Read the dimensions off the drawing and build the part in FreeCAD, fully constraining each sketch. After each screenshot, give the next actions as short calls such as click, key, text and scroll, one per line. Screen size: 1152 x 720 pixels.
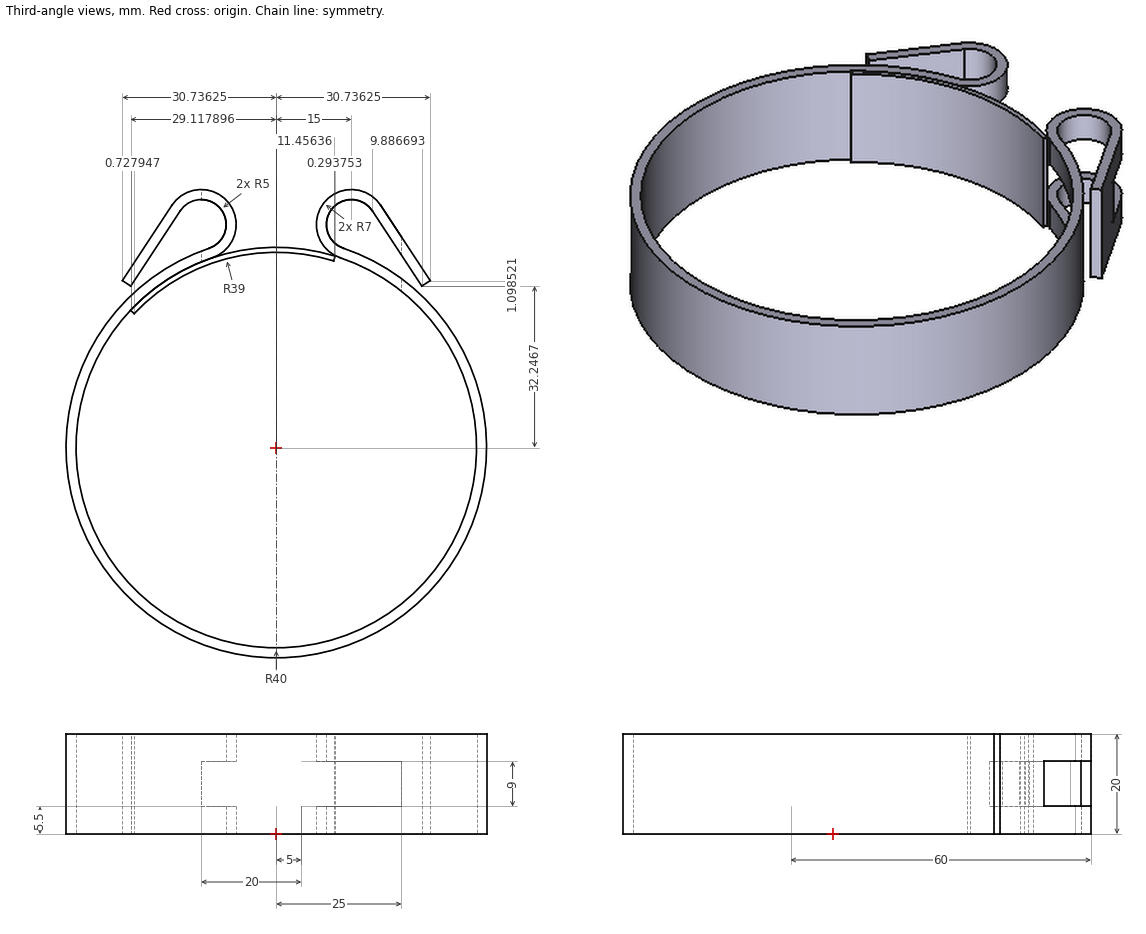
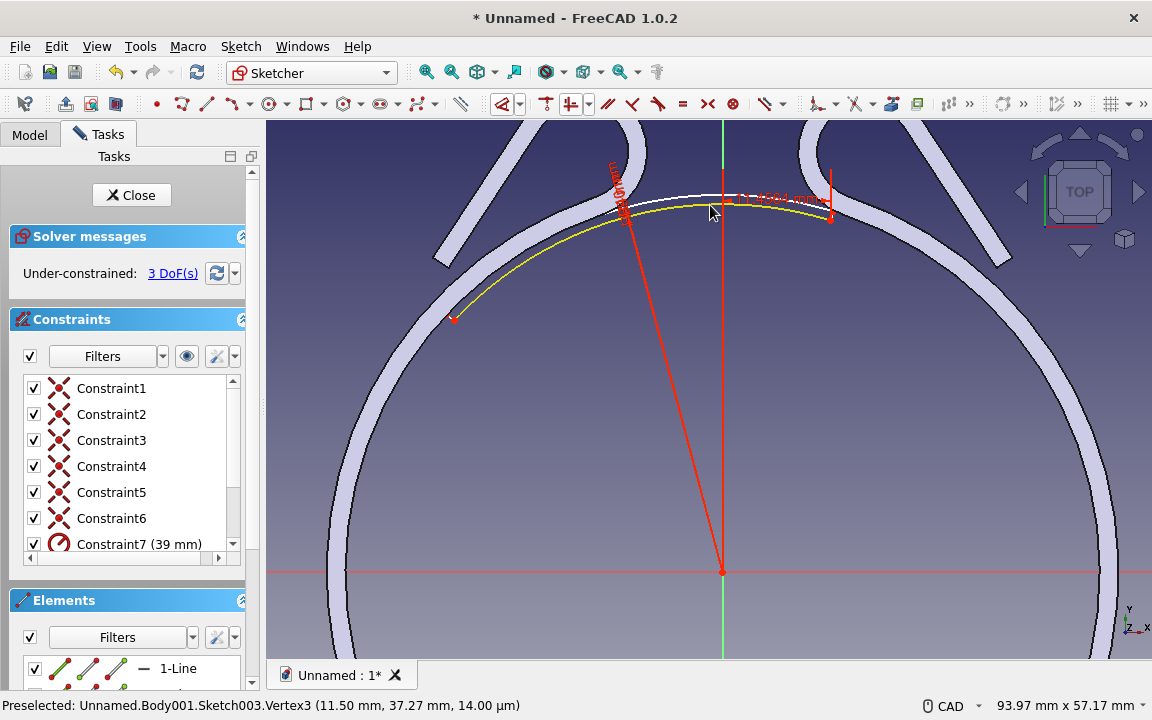
scroll(450, 318, up, 9)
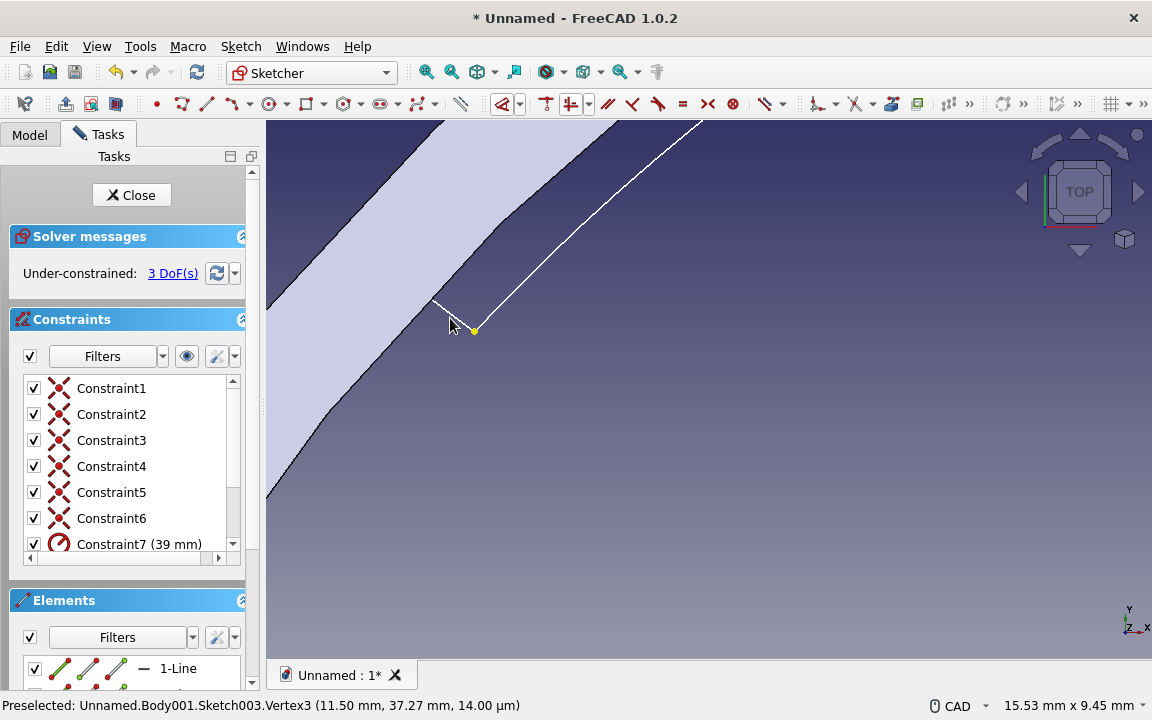
click(452, 315)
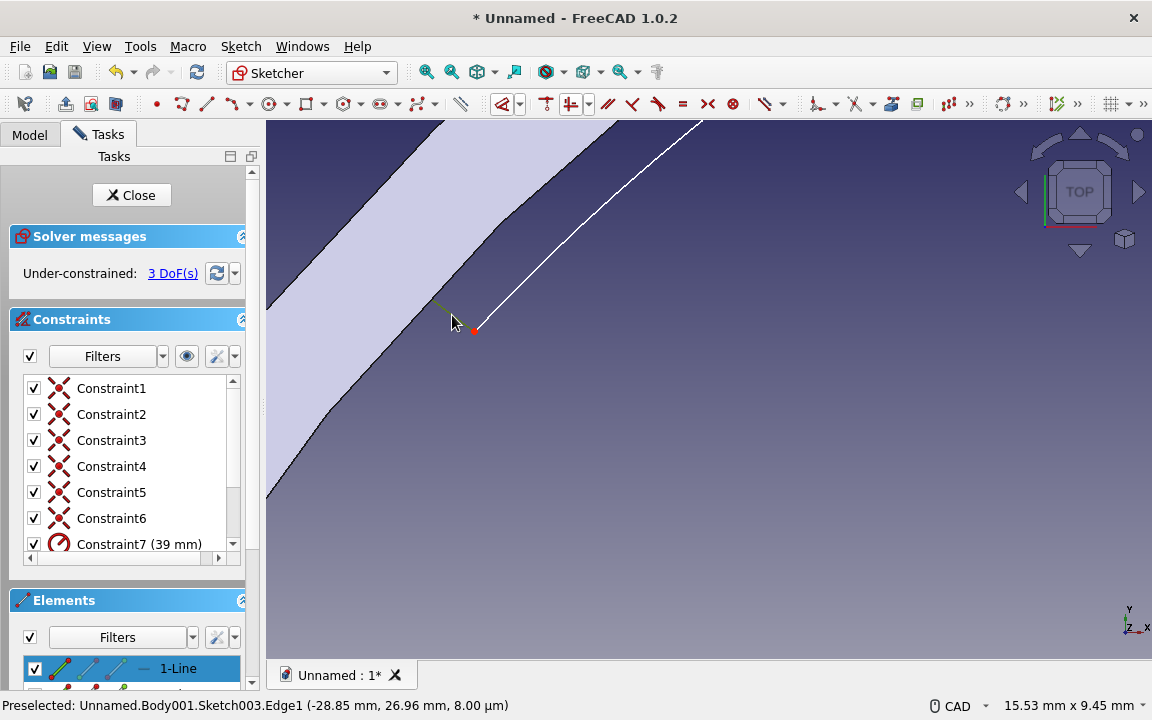
key(l)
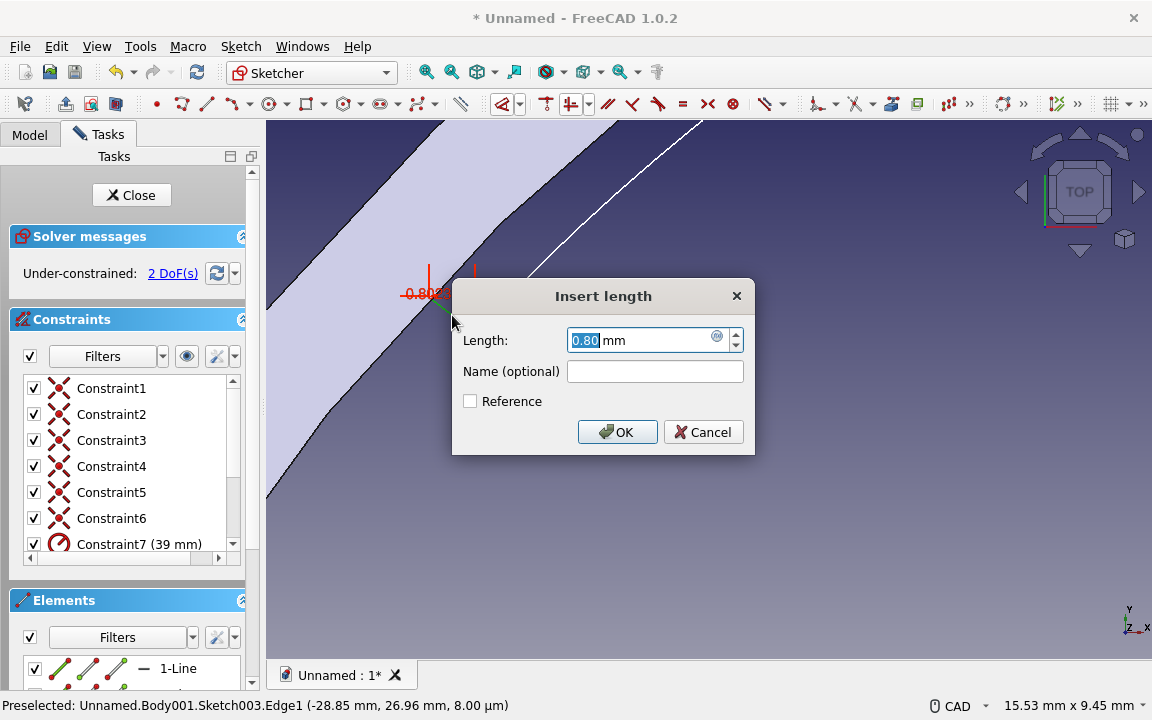
text(0.727947)
key(Return)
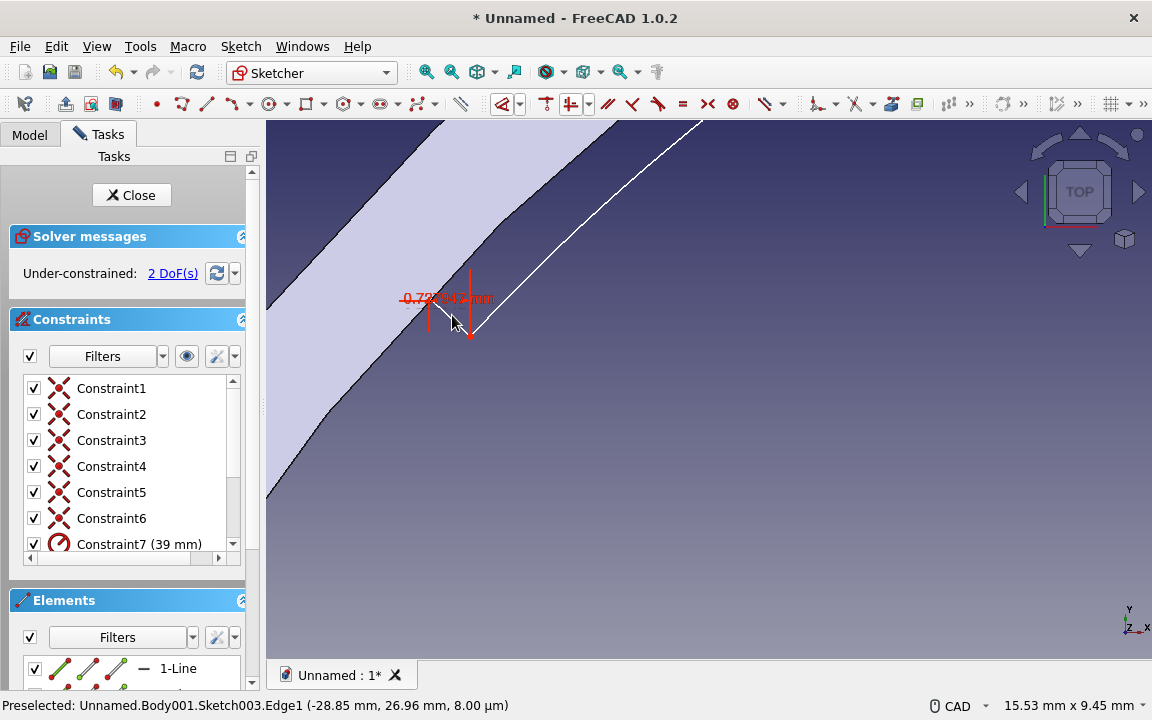
scroll(450, 318, down, 9)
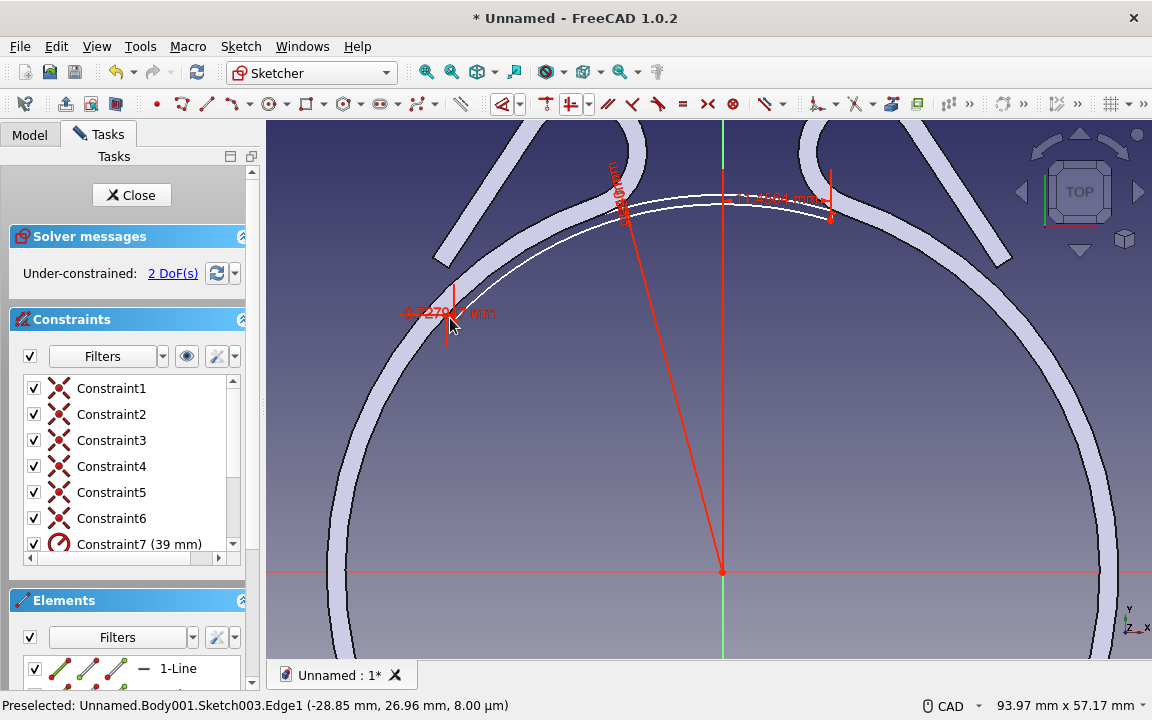
scroll(831, 218, up, 14)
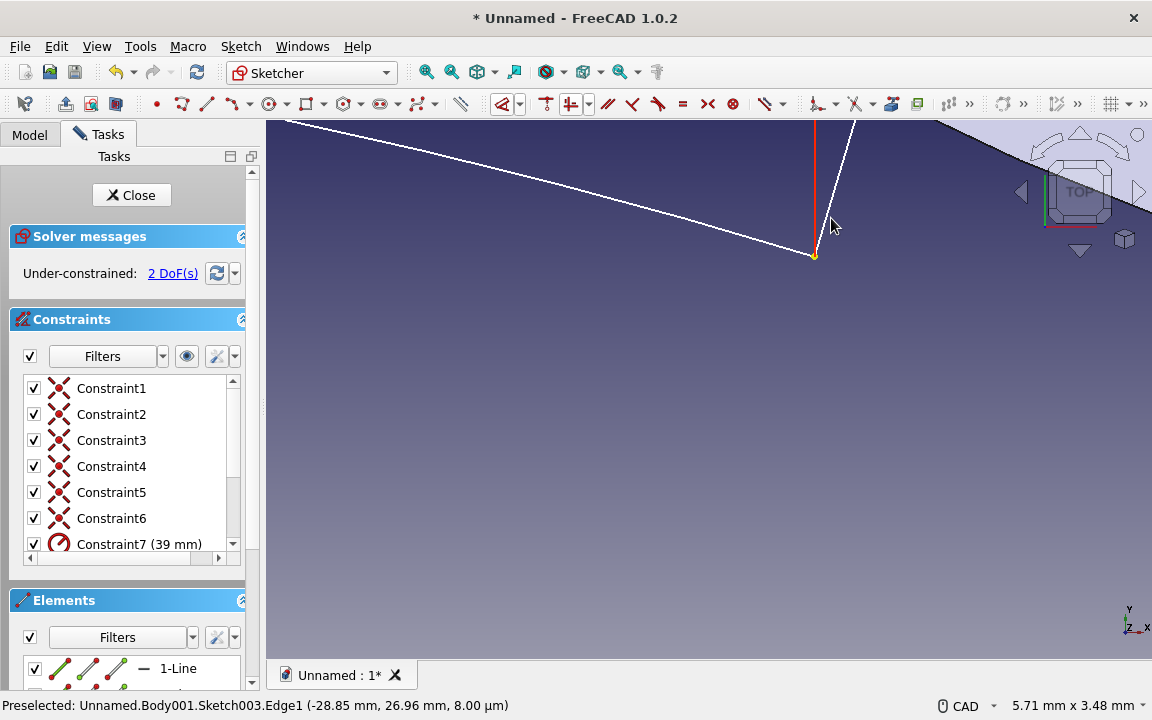
click(828, 212)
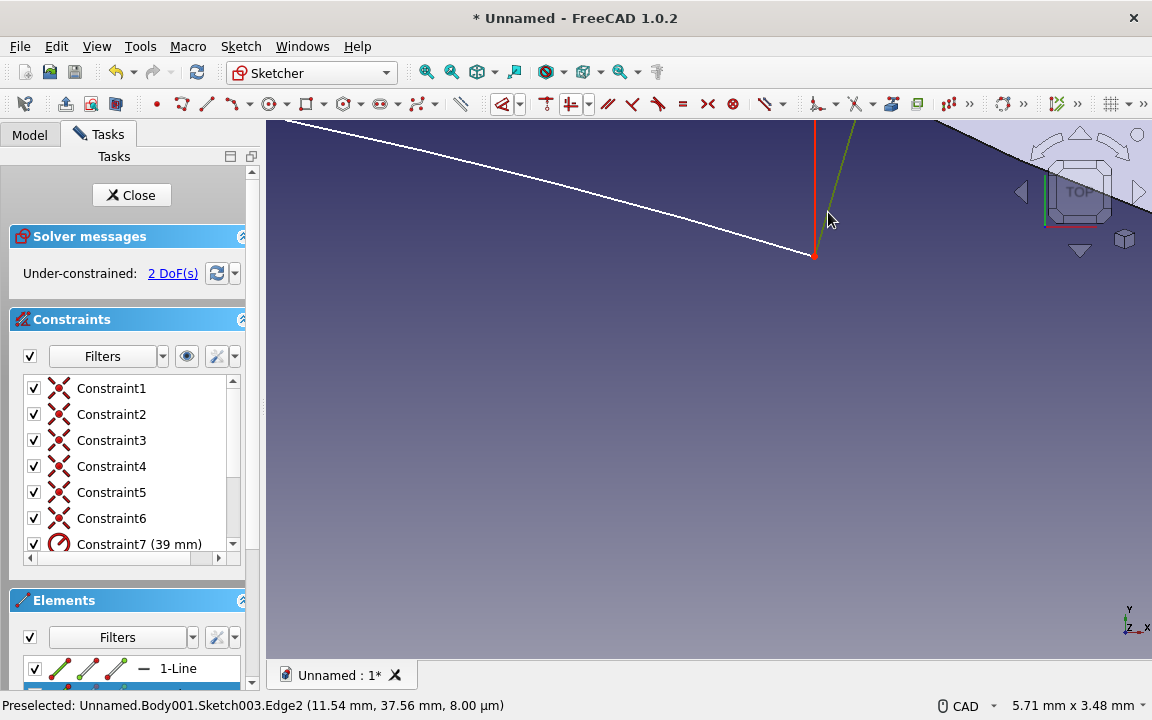
key(l)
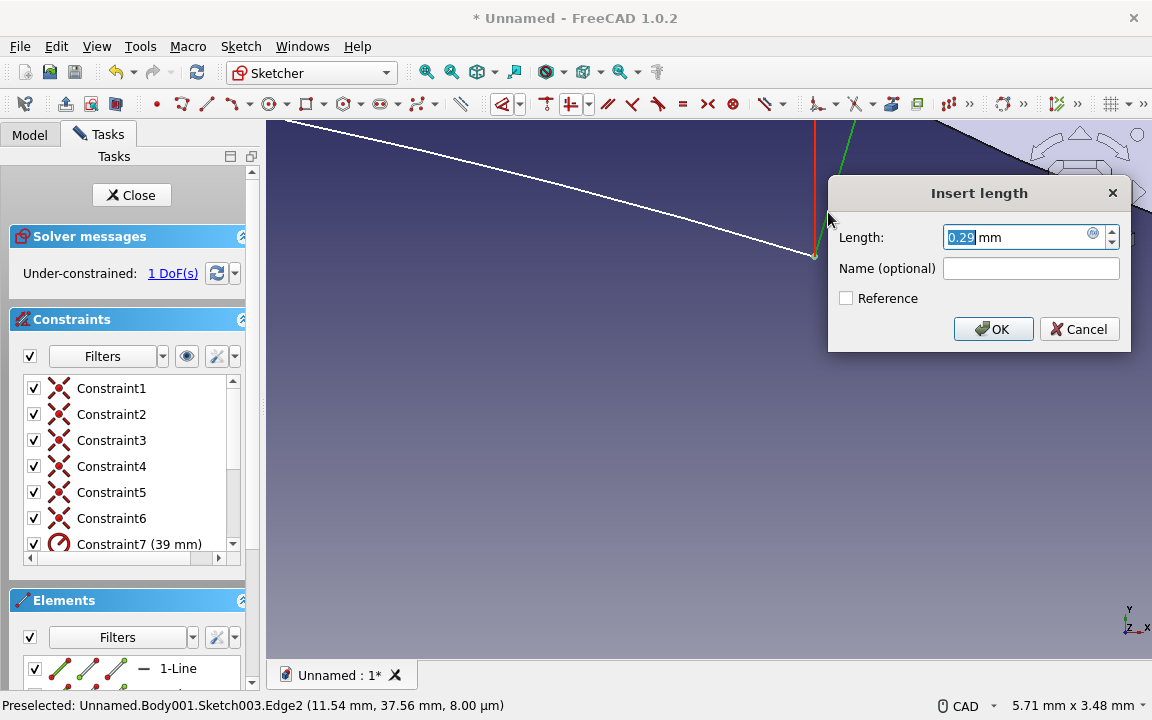
text(0.293753)
key(Return)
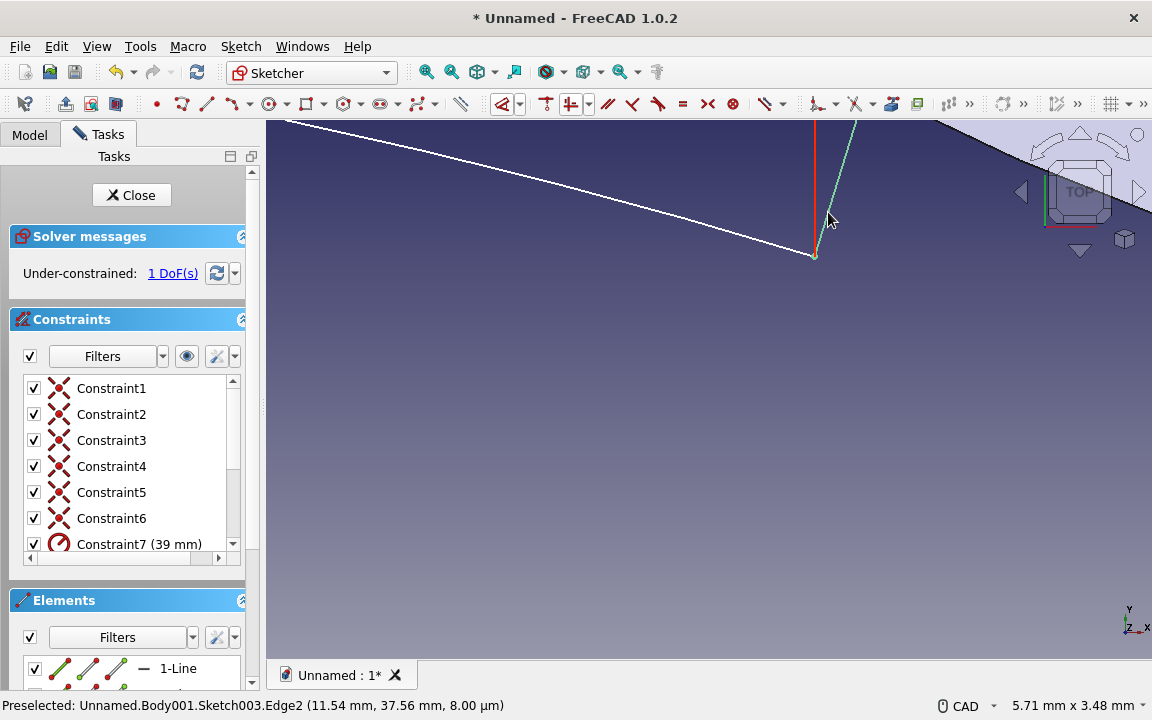
scroll(831, 218, down, 14)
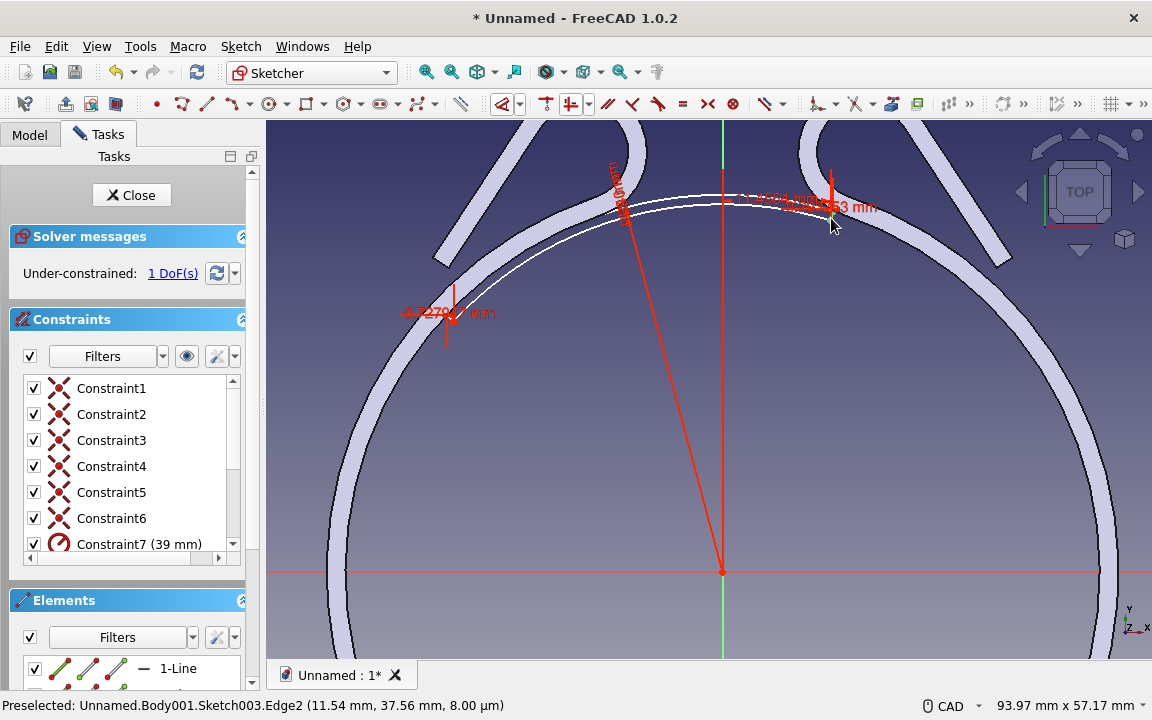
scroll(447, 315, up, 2)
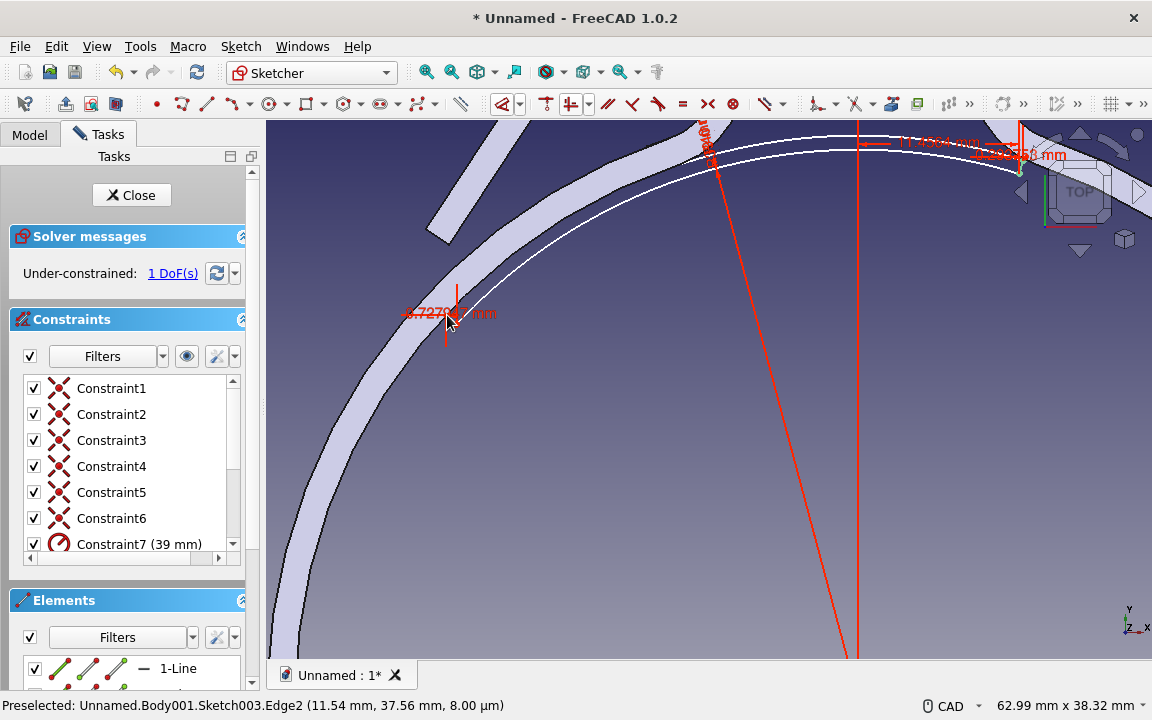
click(446, 315)